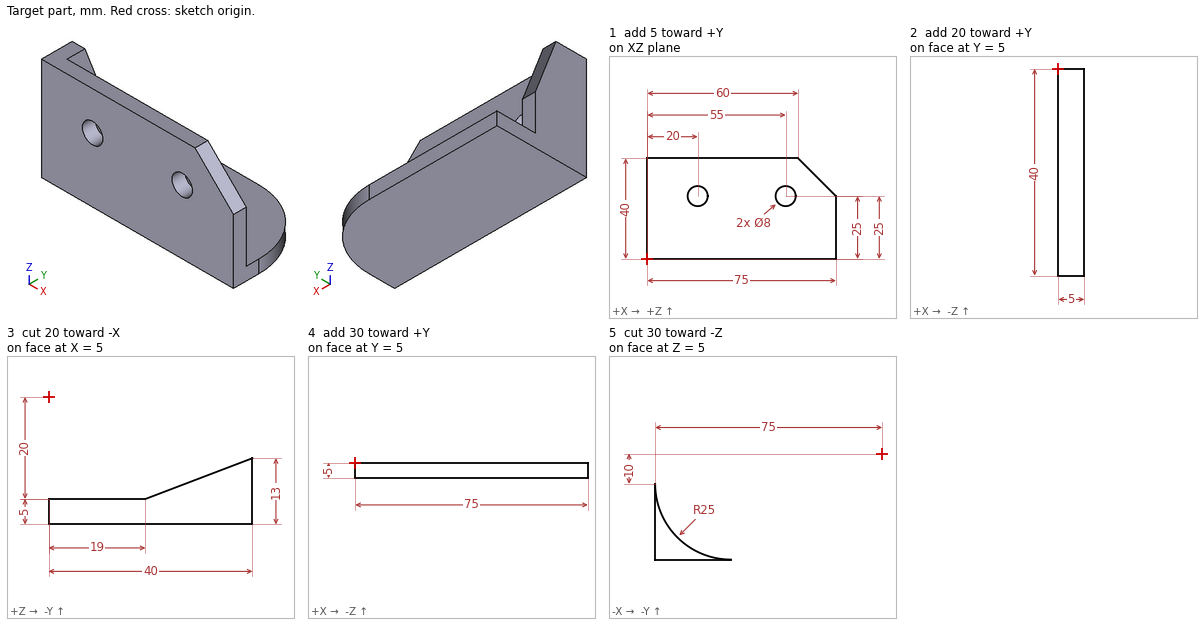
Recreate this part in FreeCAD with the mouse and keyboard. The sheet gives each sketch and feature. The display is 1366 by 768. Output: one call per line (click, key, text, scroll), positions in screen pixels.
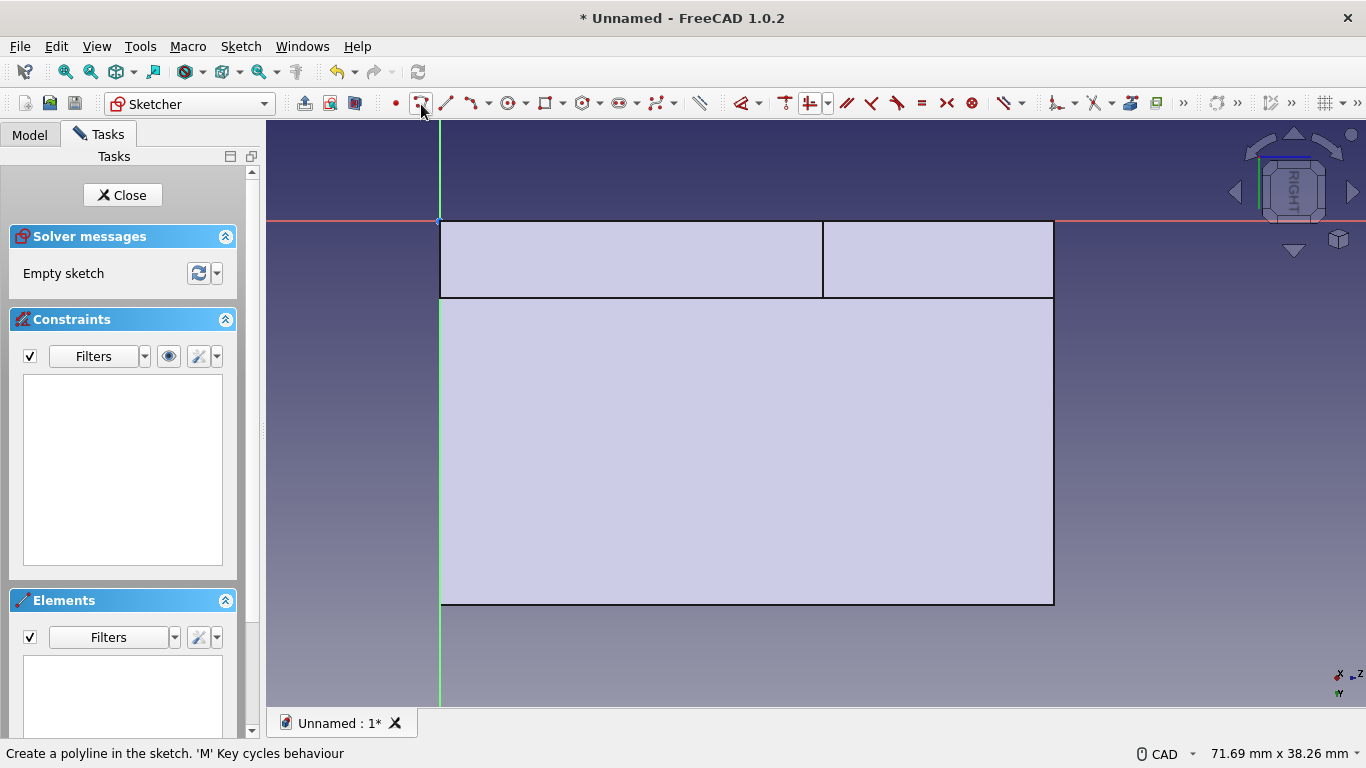
click(440, 528)
click(449, 605)
click(1054, 605)
click(1054, 405)
click(731, 528)
click(440, 529)
key(Escape)
key(Escape)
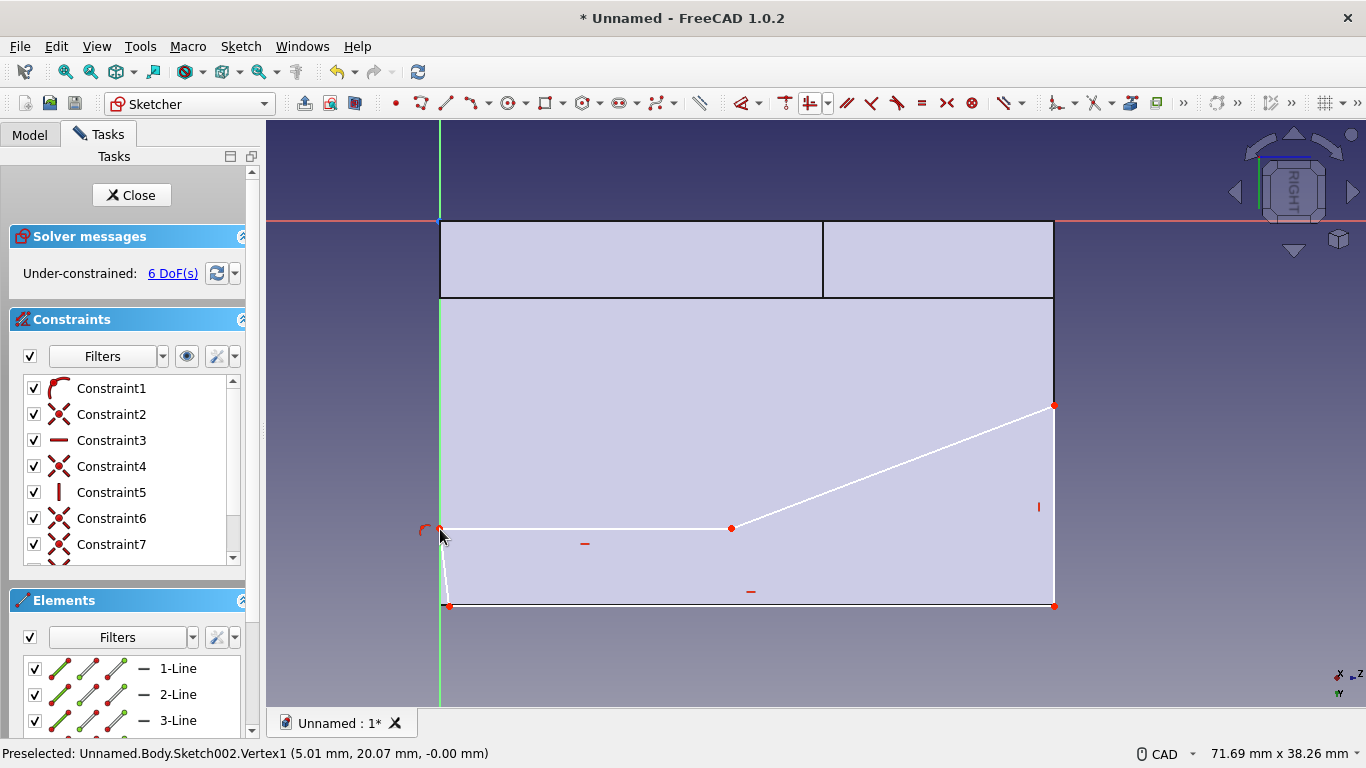
click(443, 552)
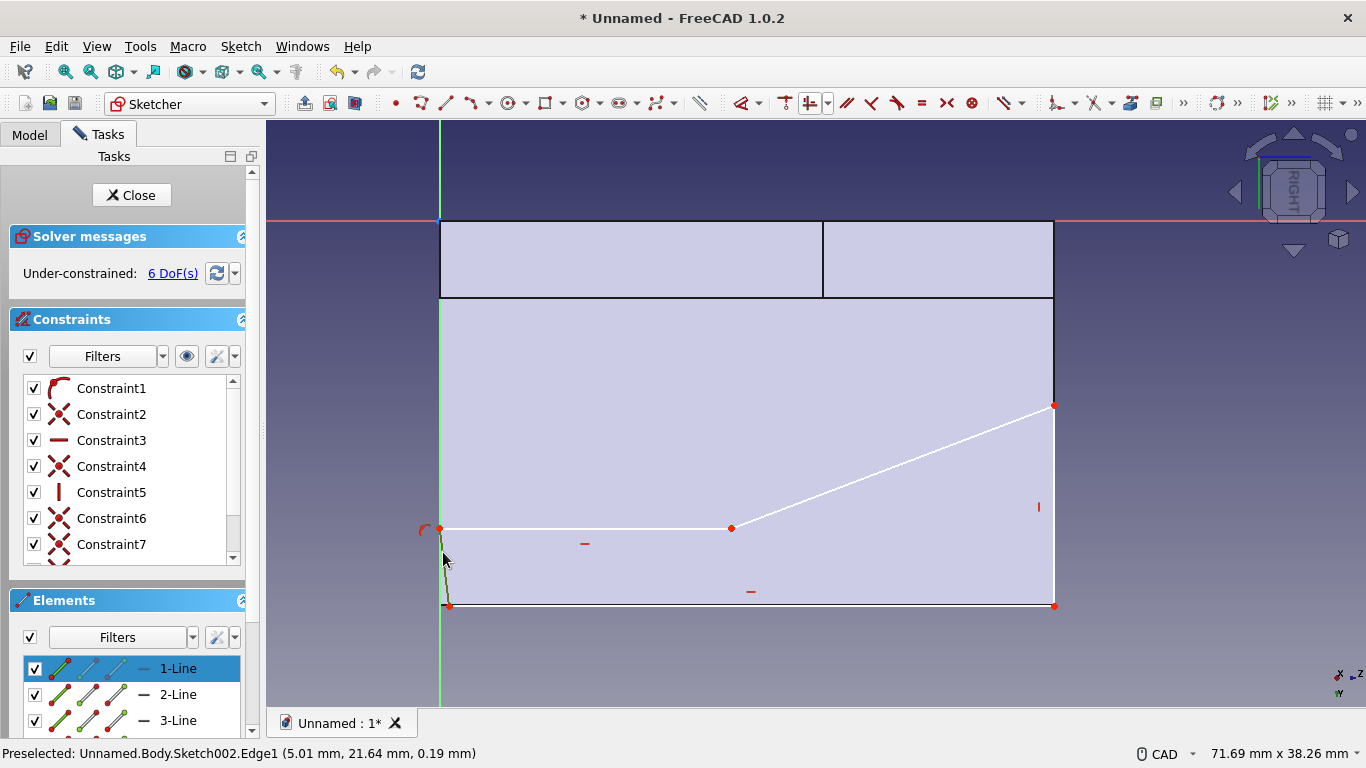
key(v)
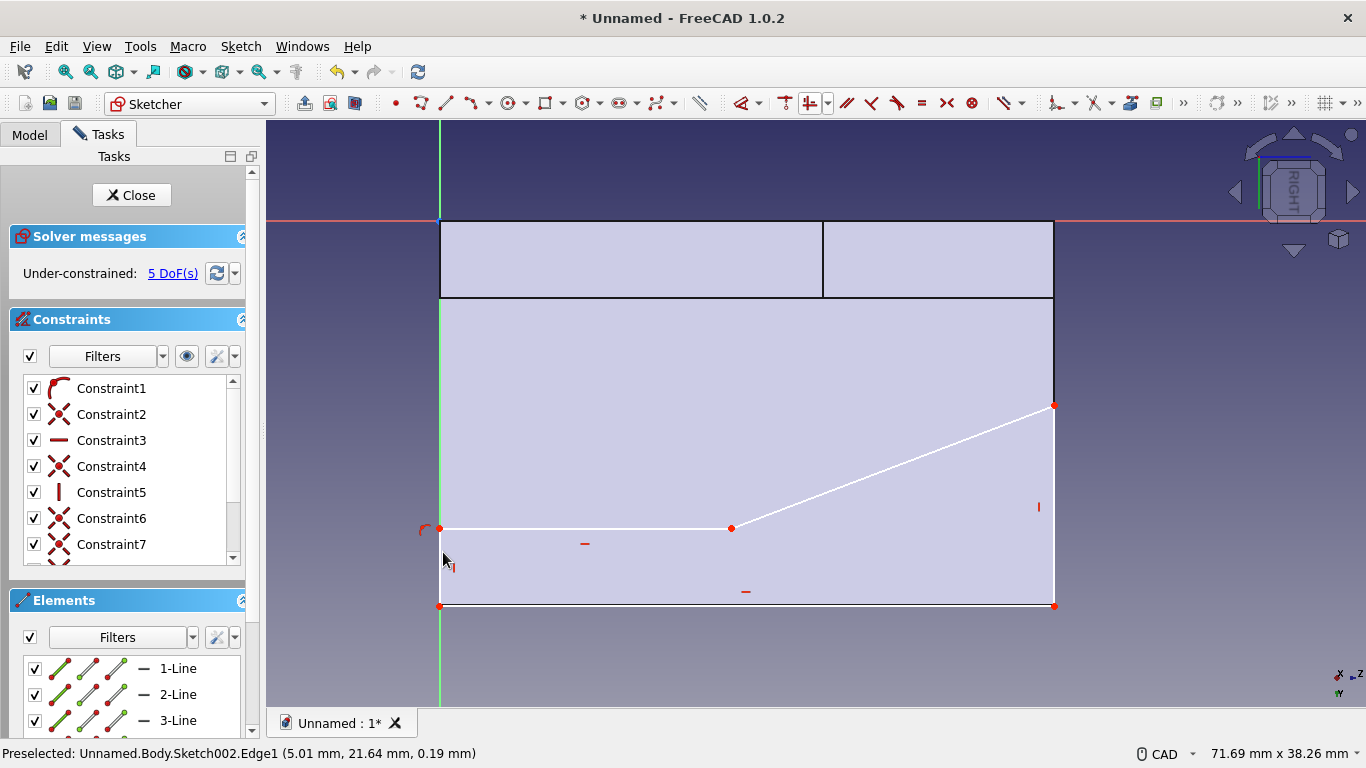
click(740, 104)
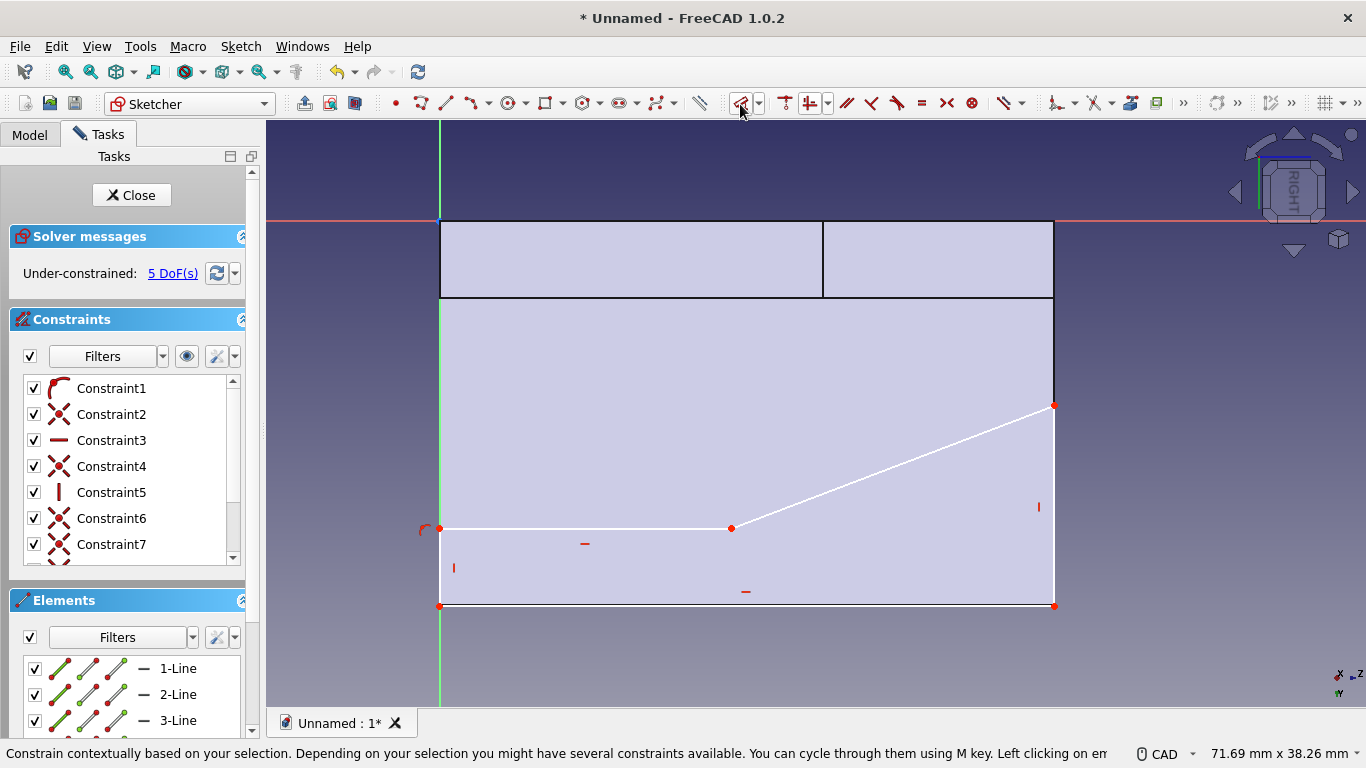
click(440, 552)
click(406, 568)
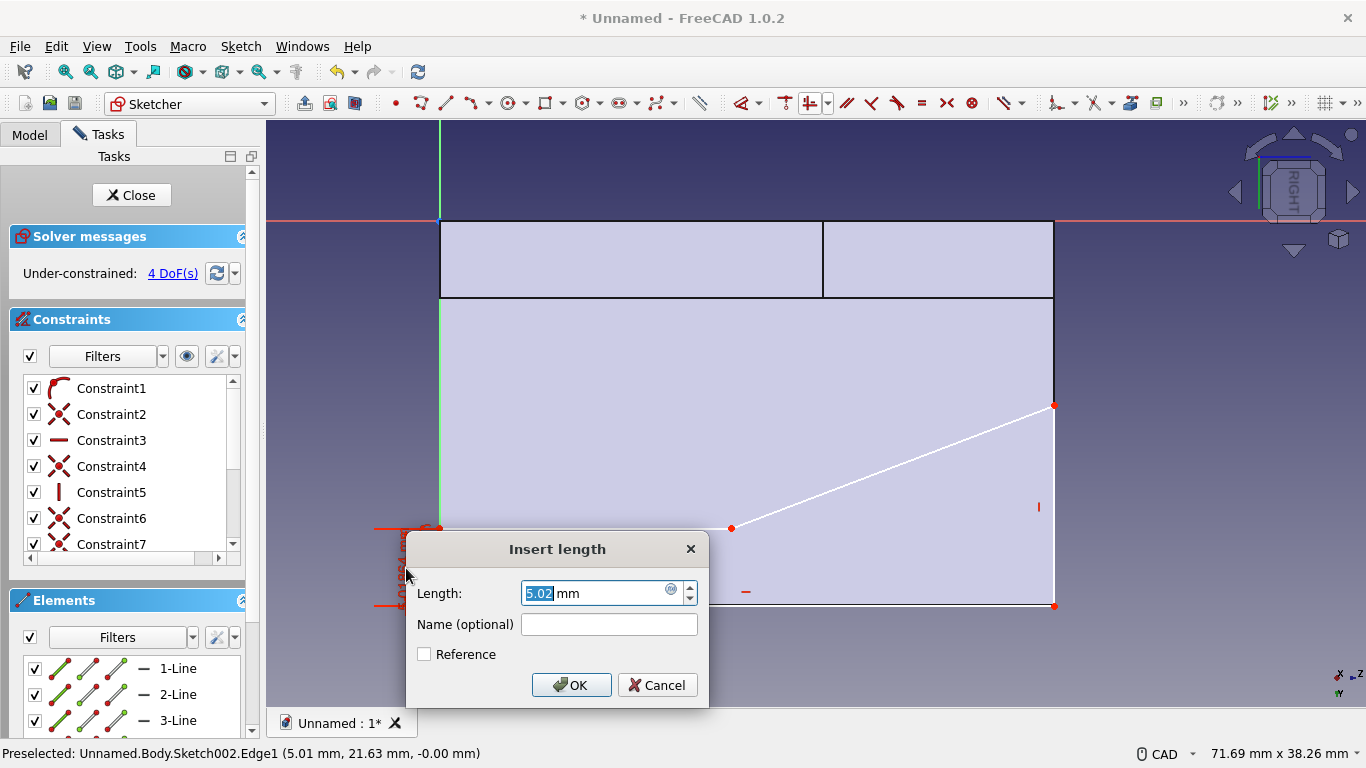
text(5)
key(Return)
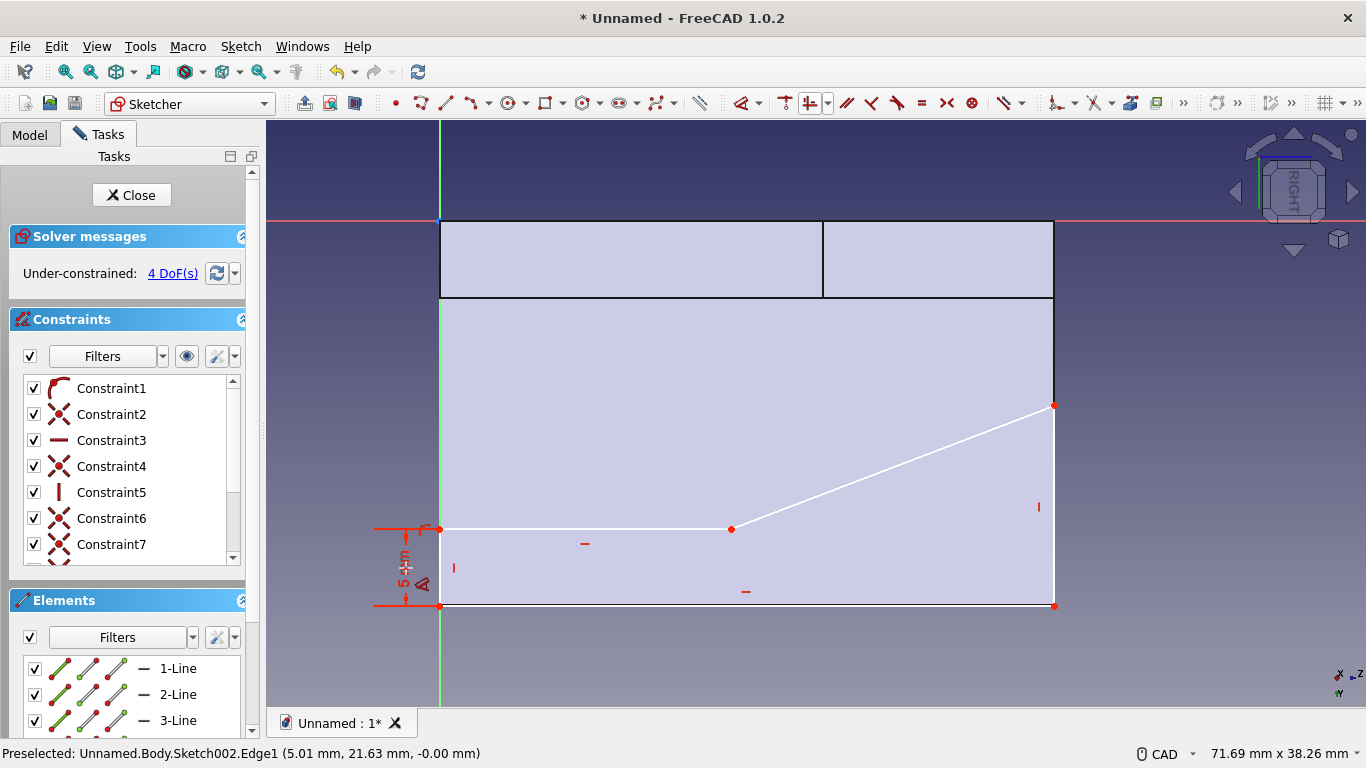
click(624, 606)
click(747, 640)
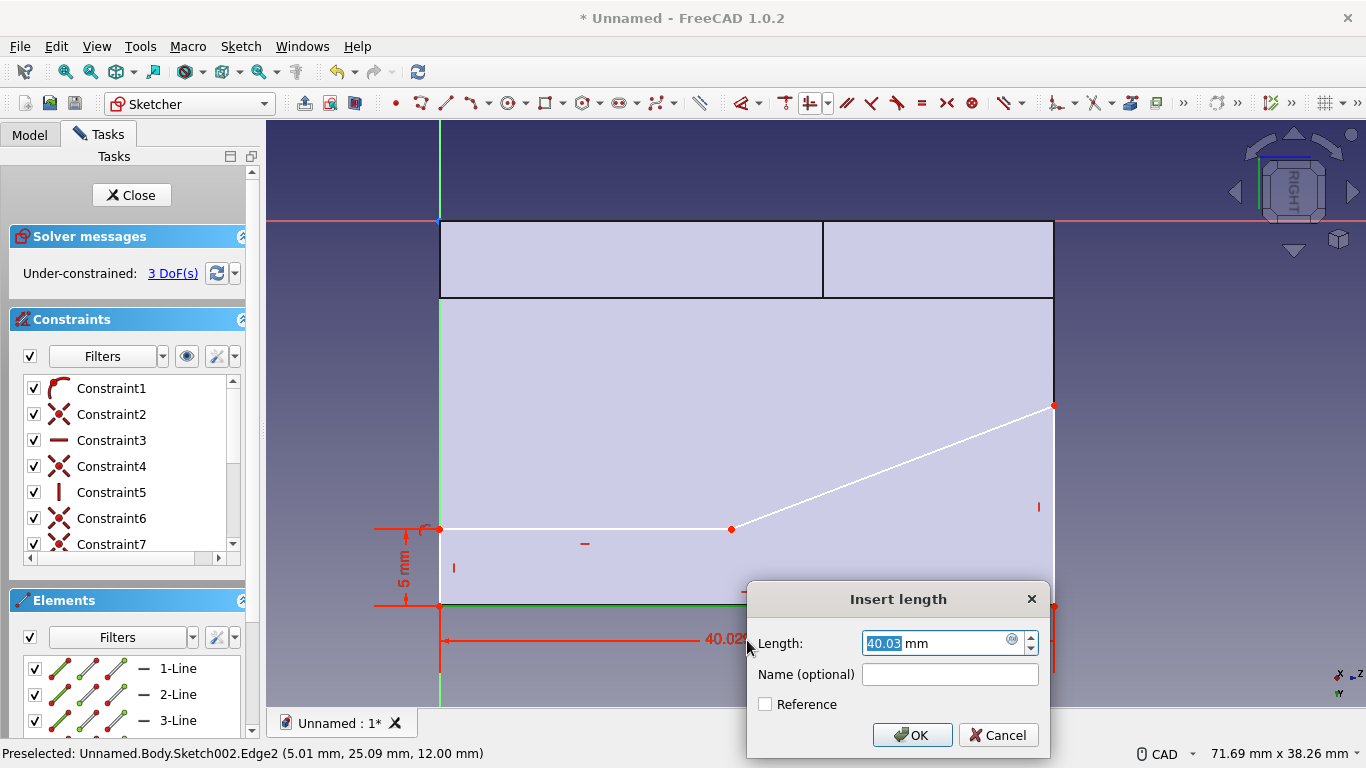
text(40)
key(Return)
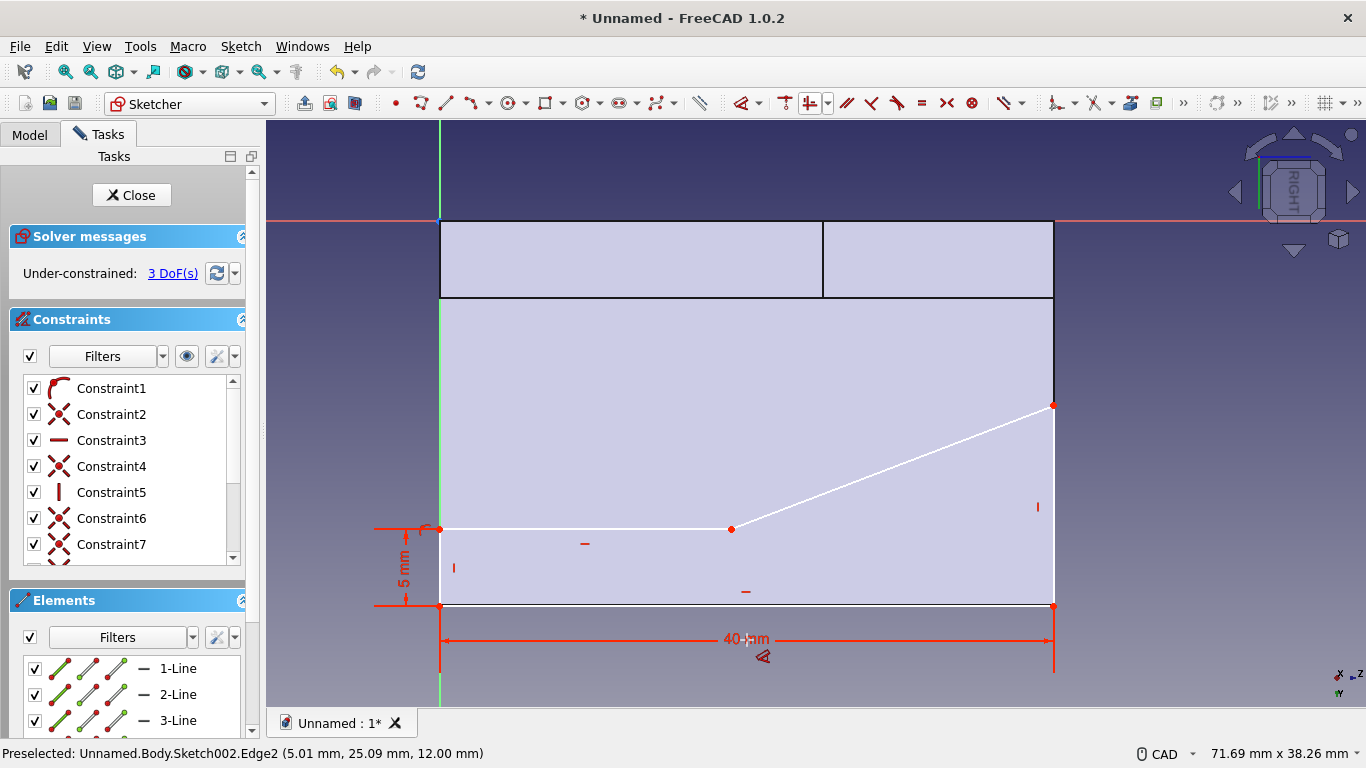
click(1054, 546)
click(1088, 506)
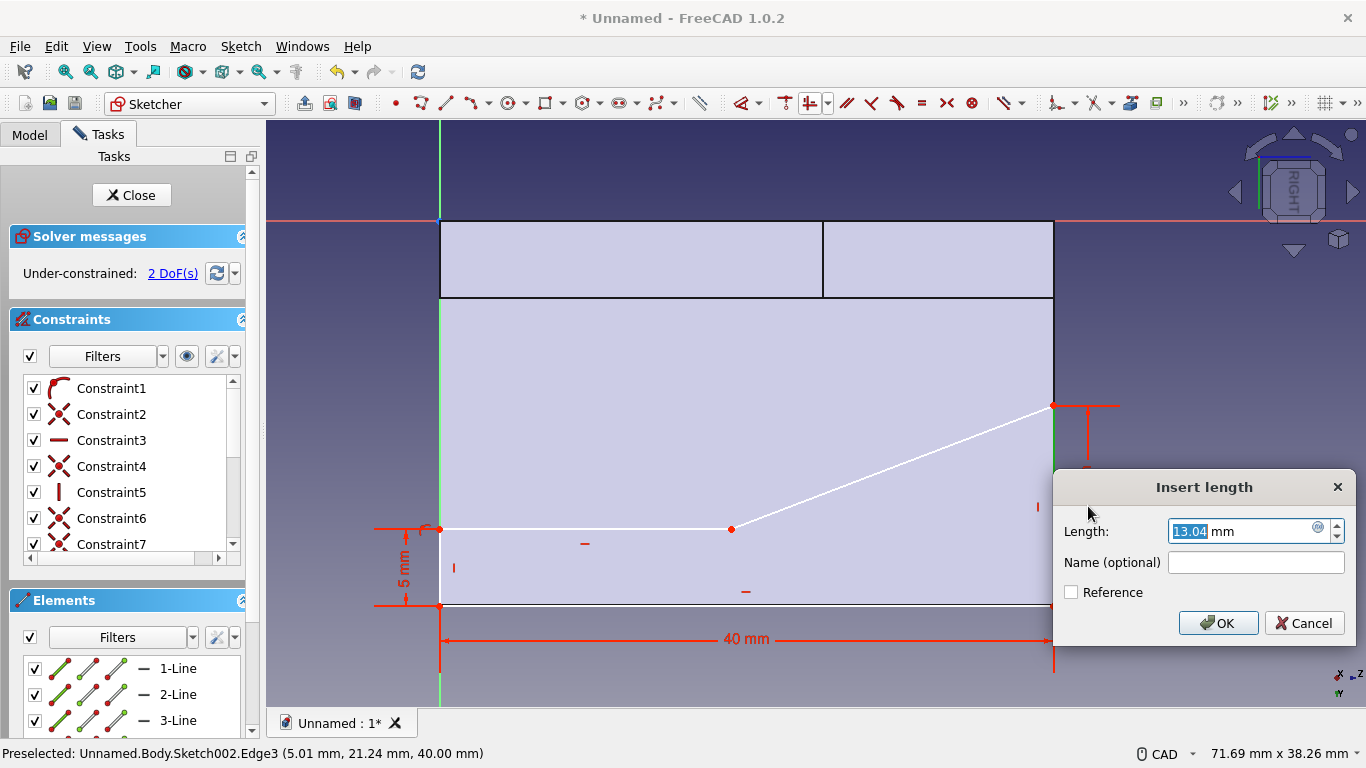
text(13)
key(Return)